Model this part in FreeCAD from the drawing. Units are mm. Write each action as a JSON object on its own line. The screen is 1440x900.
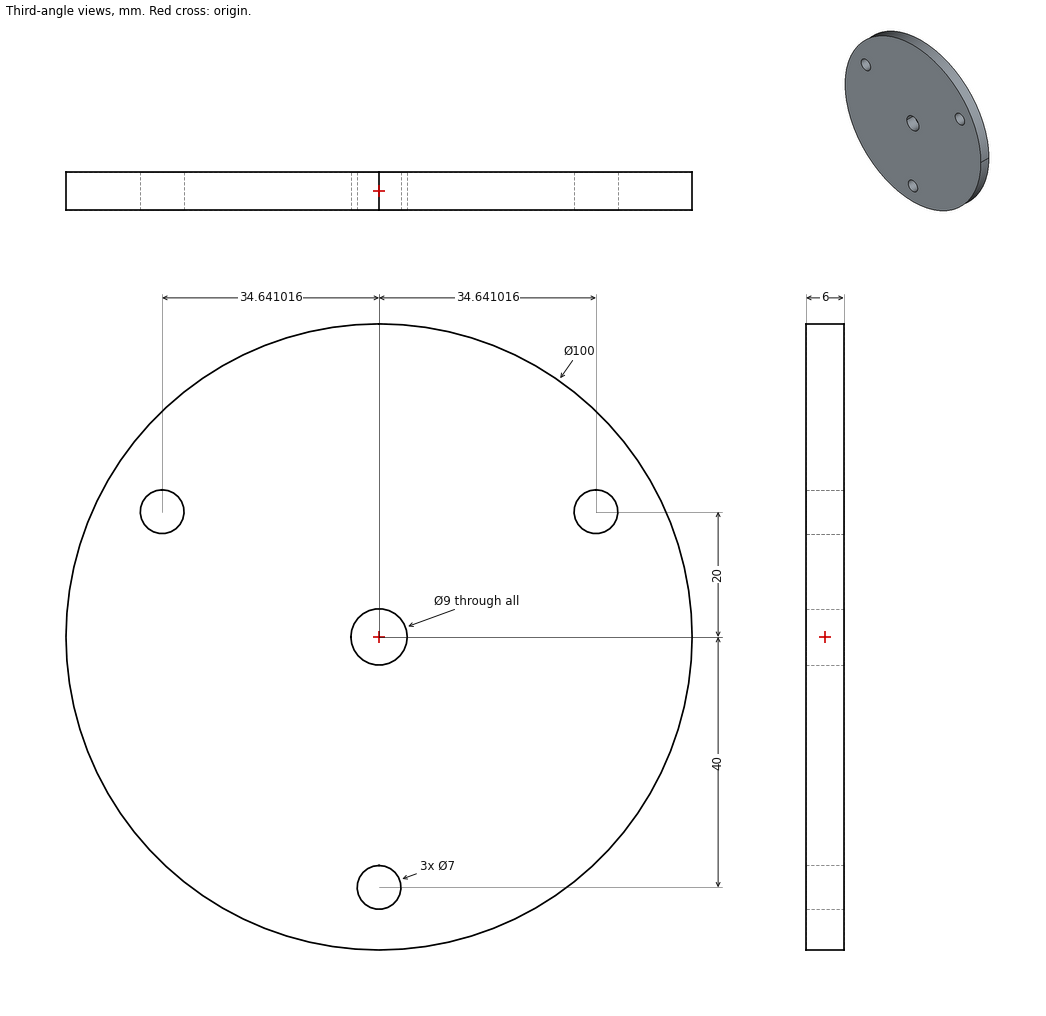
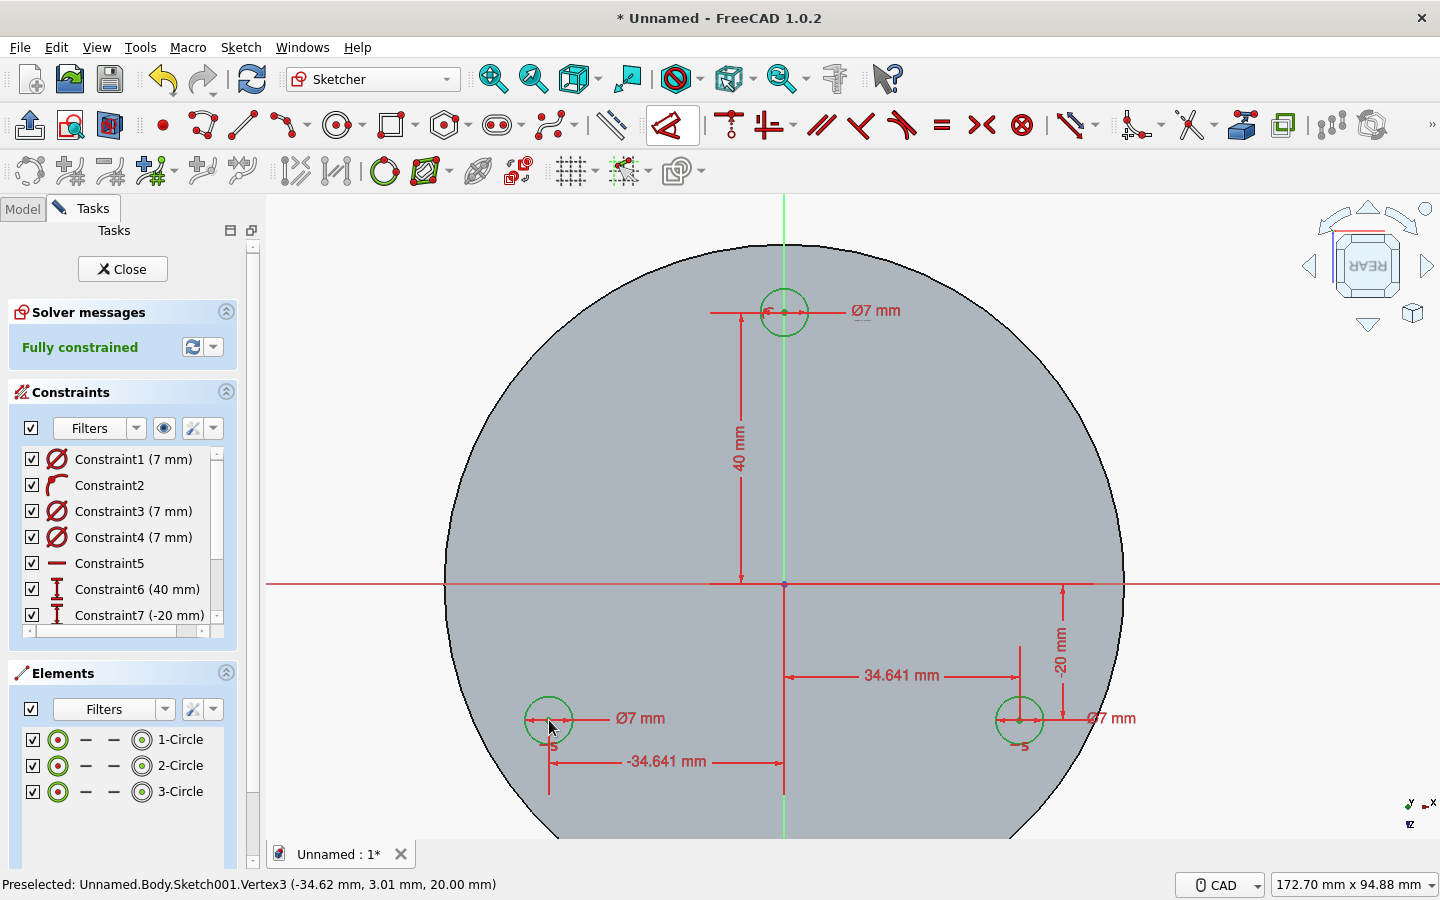
{"action": "left_click", "coordinate": [123, 269]}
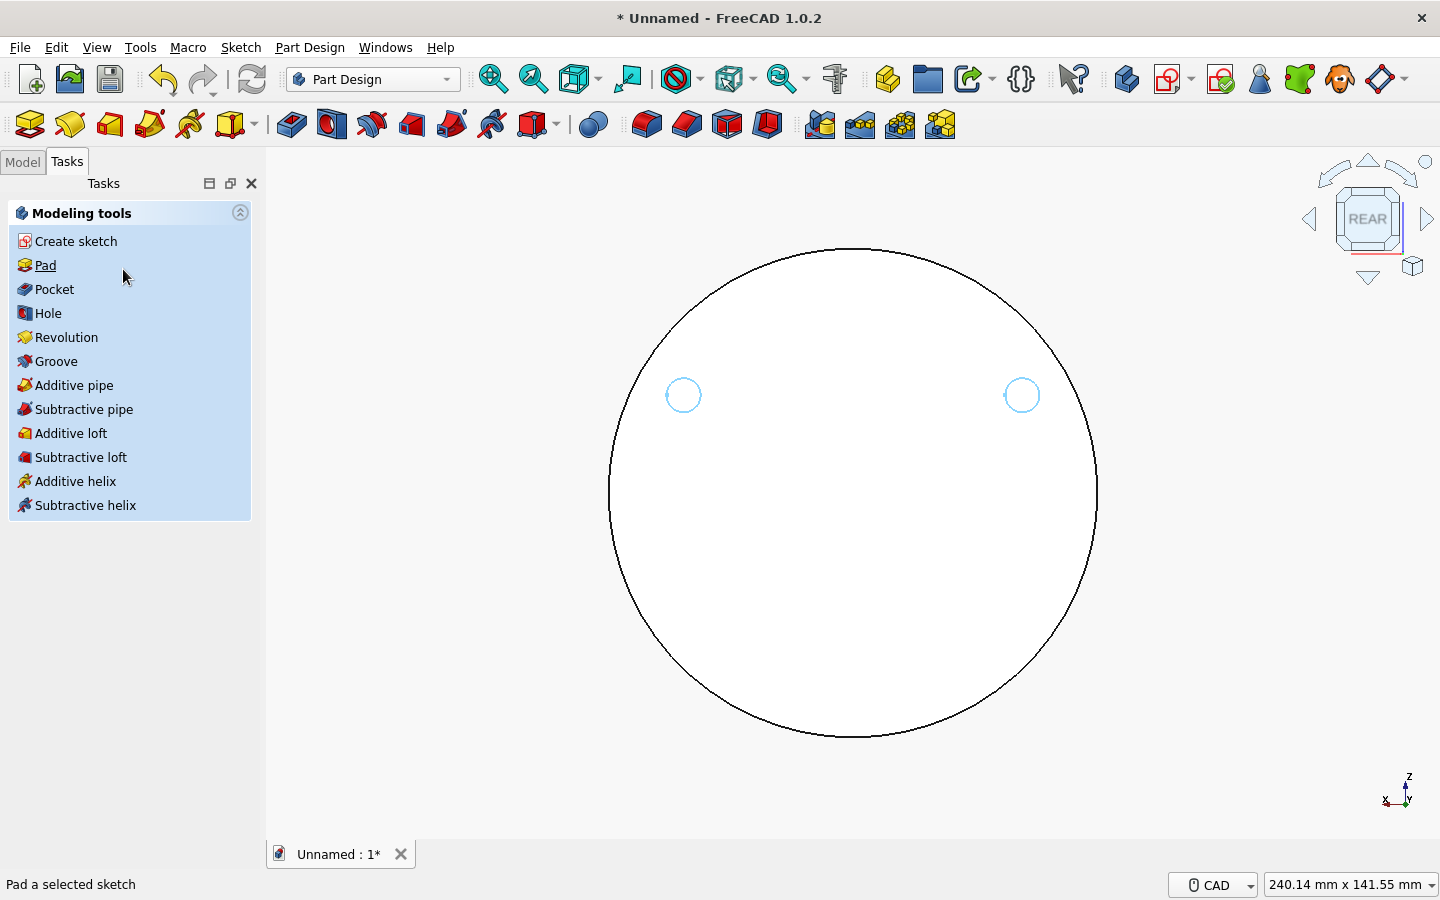
{"action": "left_click", "coordinate": [292, 124]}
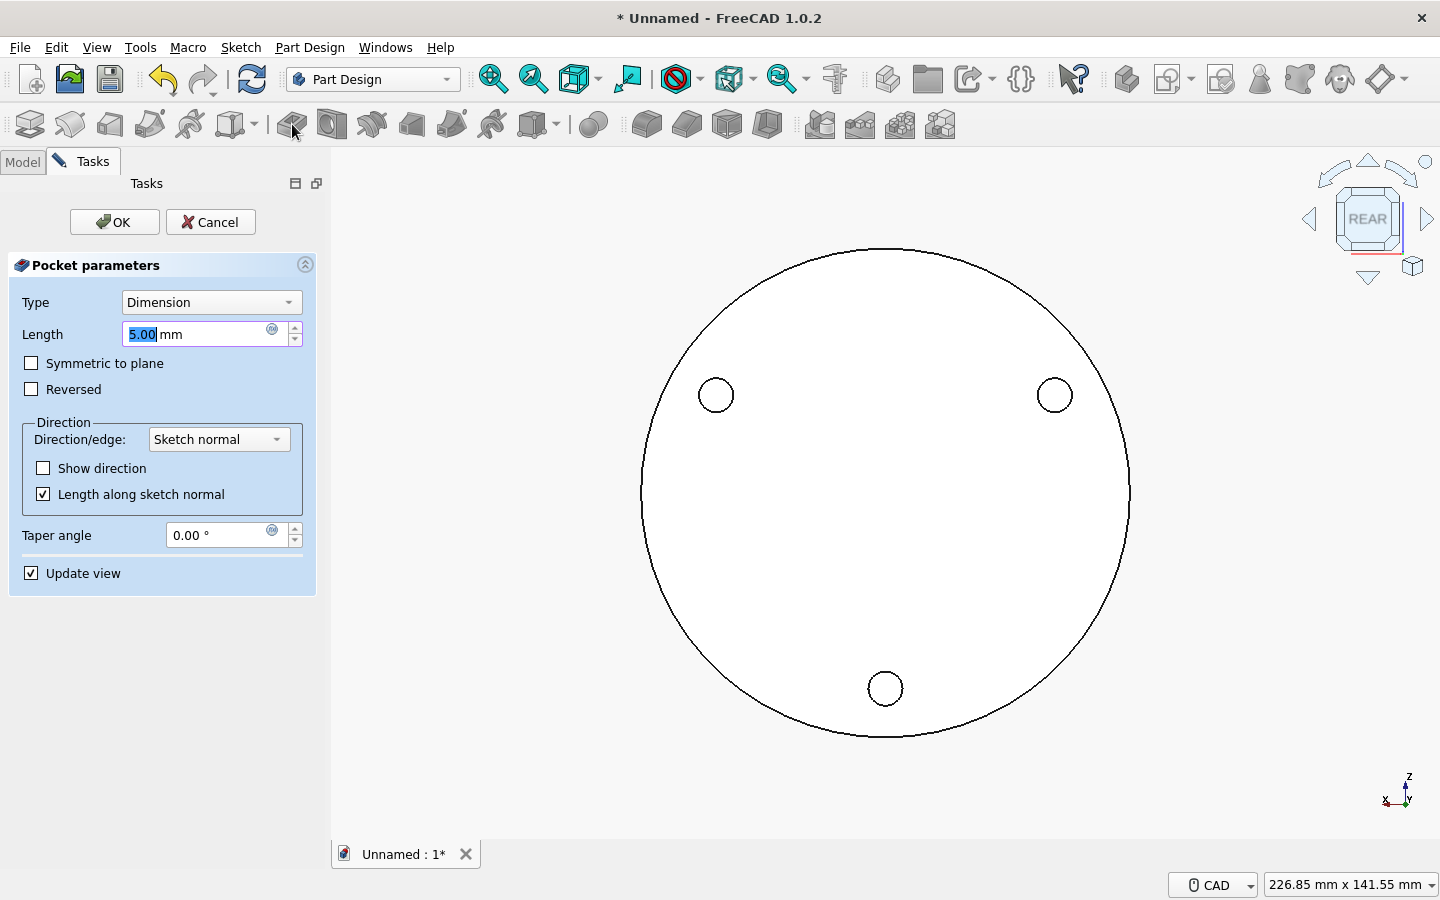
{"action": "left_click", "coordinate": [212, 302]}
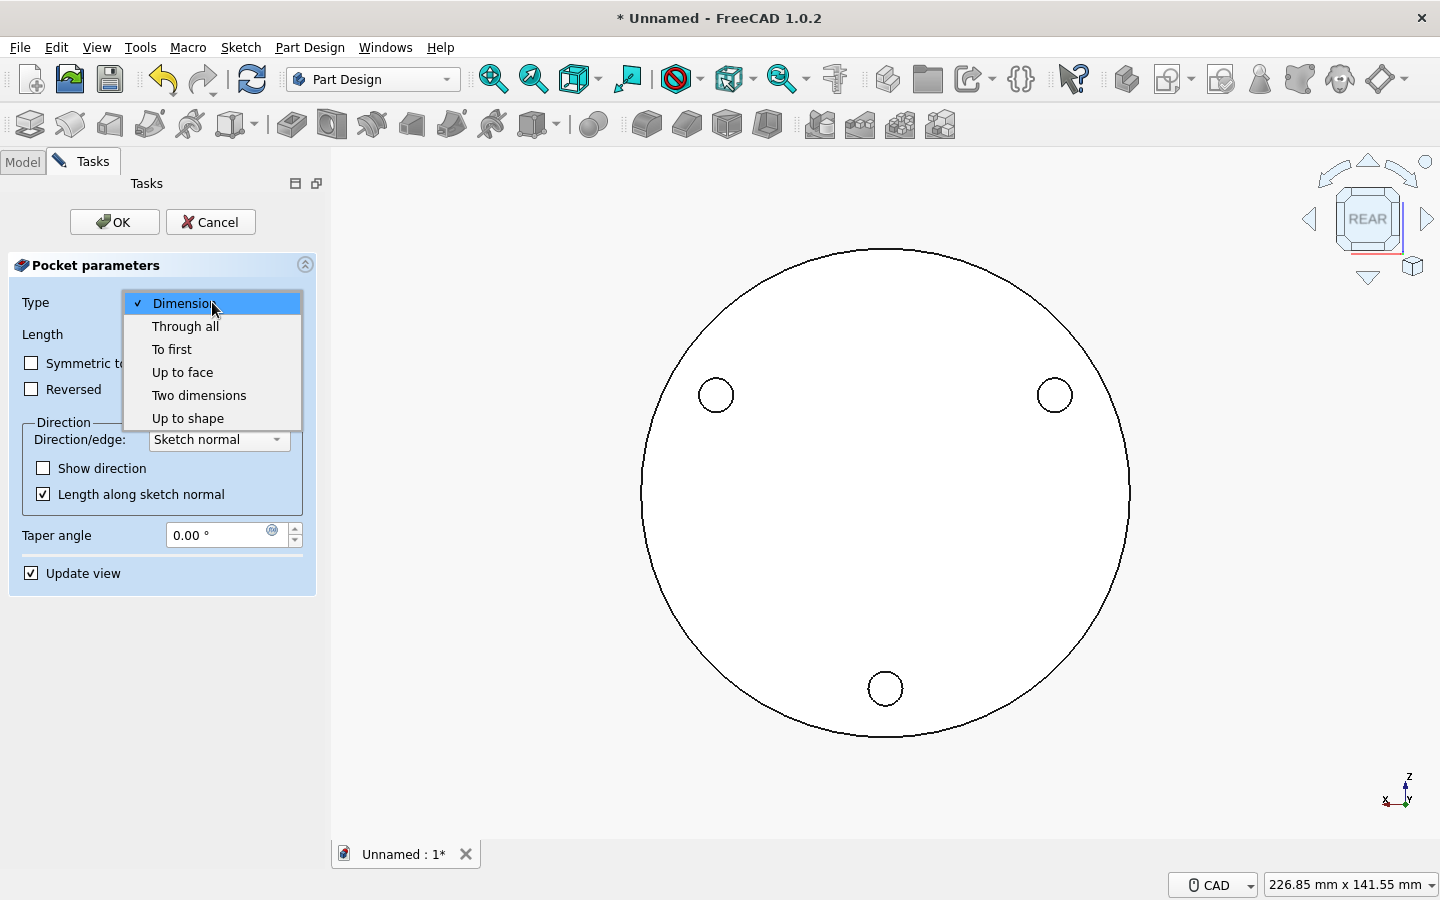
{"action": "left_click", "coordinate": [212, 326]}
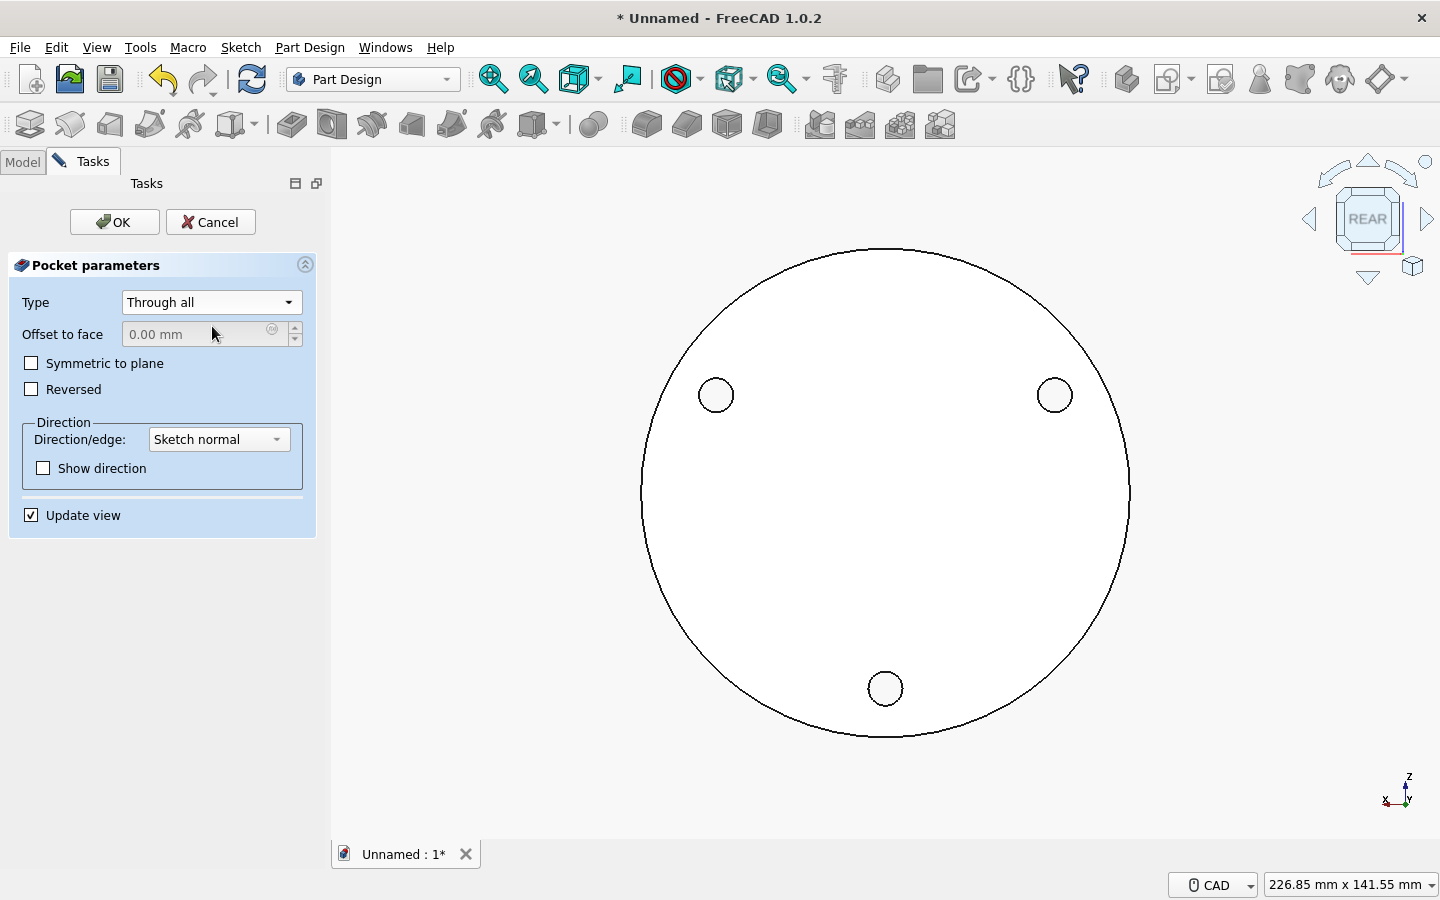
{"action": "left_click", "coordinate": [115, 222]}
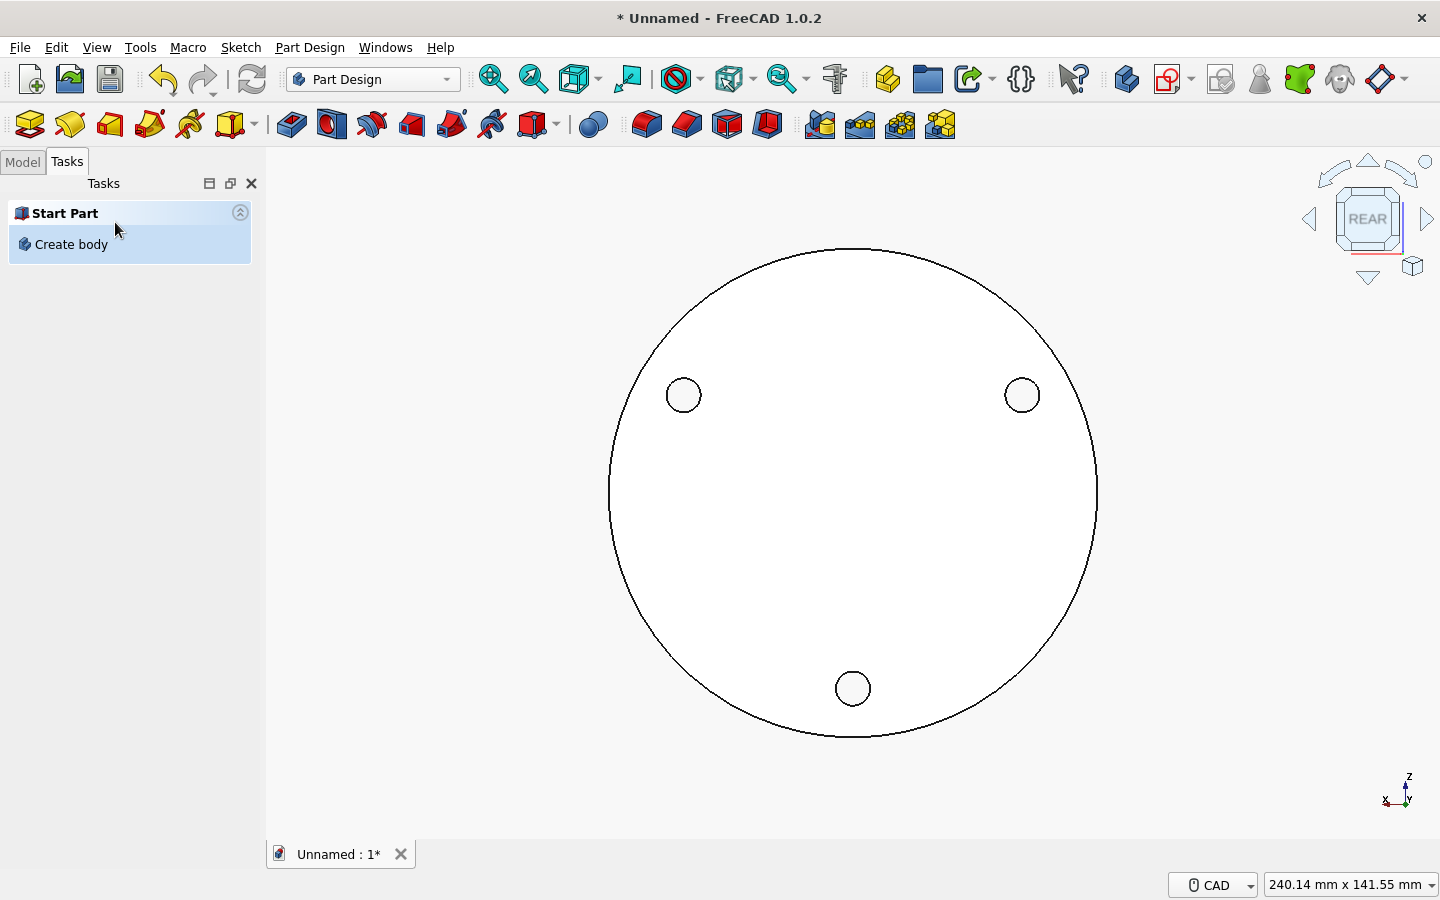
{"action": "left_click", "coordinate": [853, 492]}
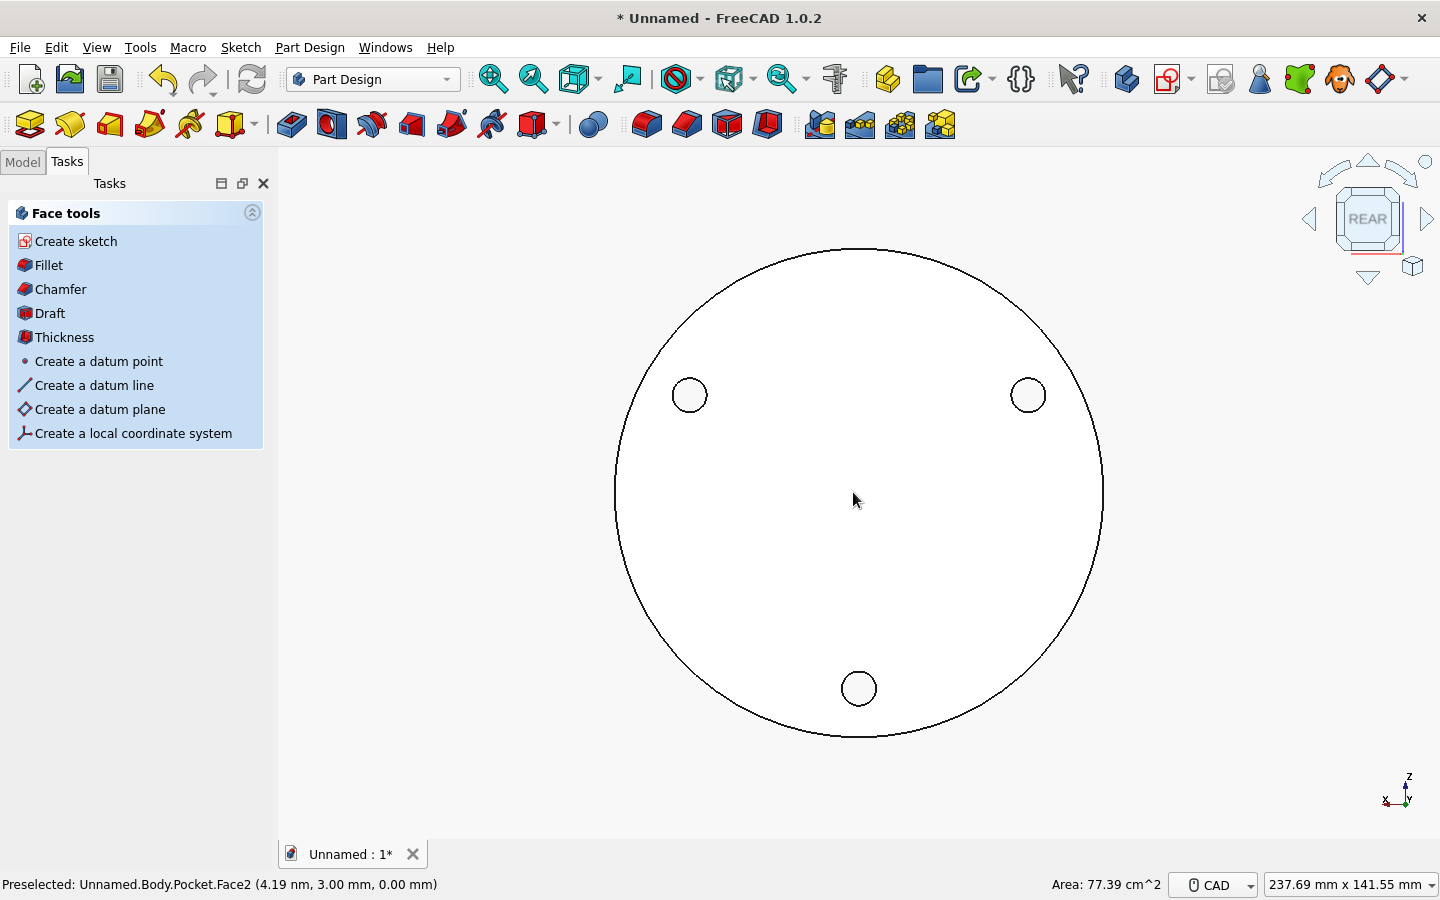
{"action": "left_click", "coordinate": [1168, 80]}